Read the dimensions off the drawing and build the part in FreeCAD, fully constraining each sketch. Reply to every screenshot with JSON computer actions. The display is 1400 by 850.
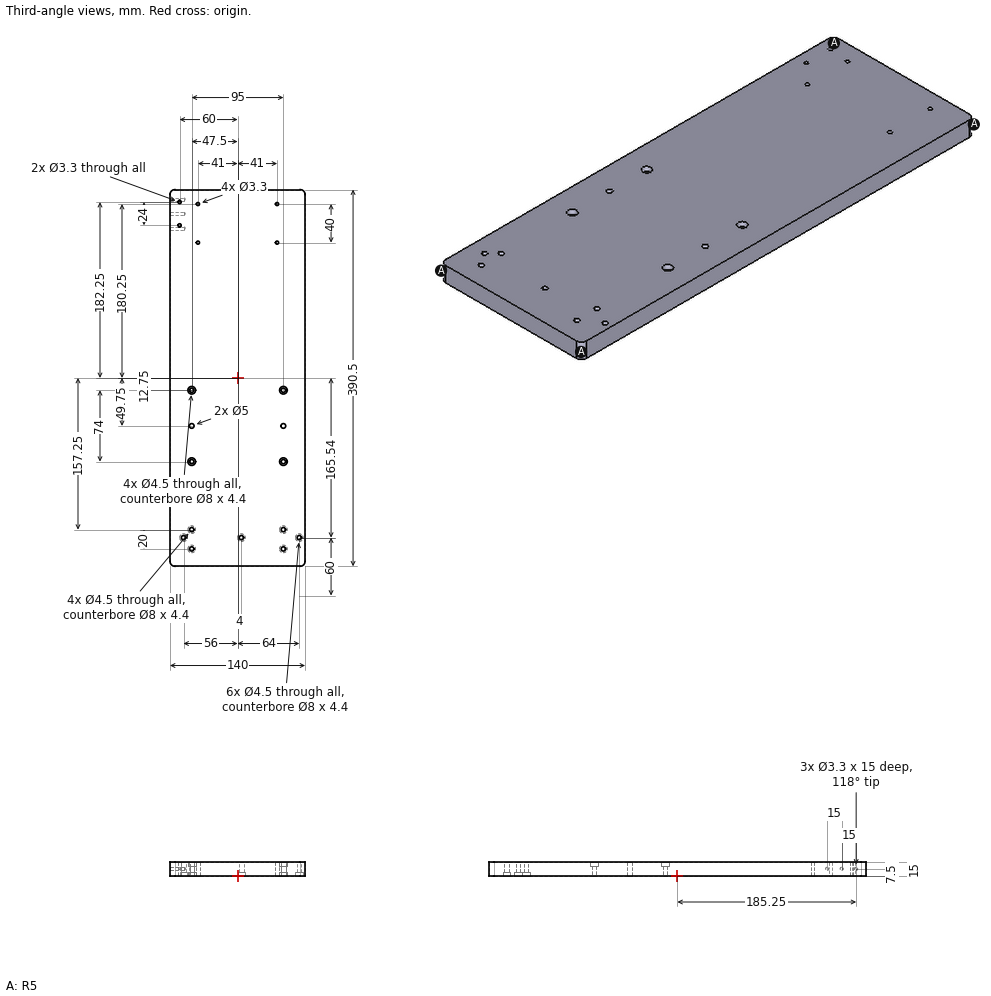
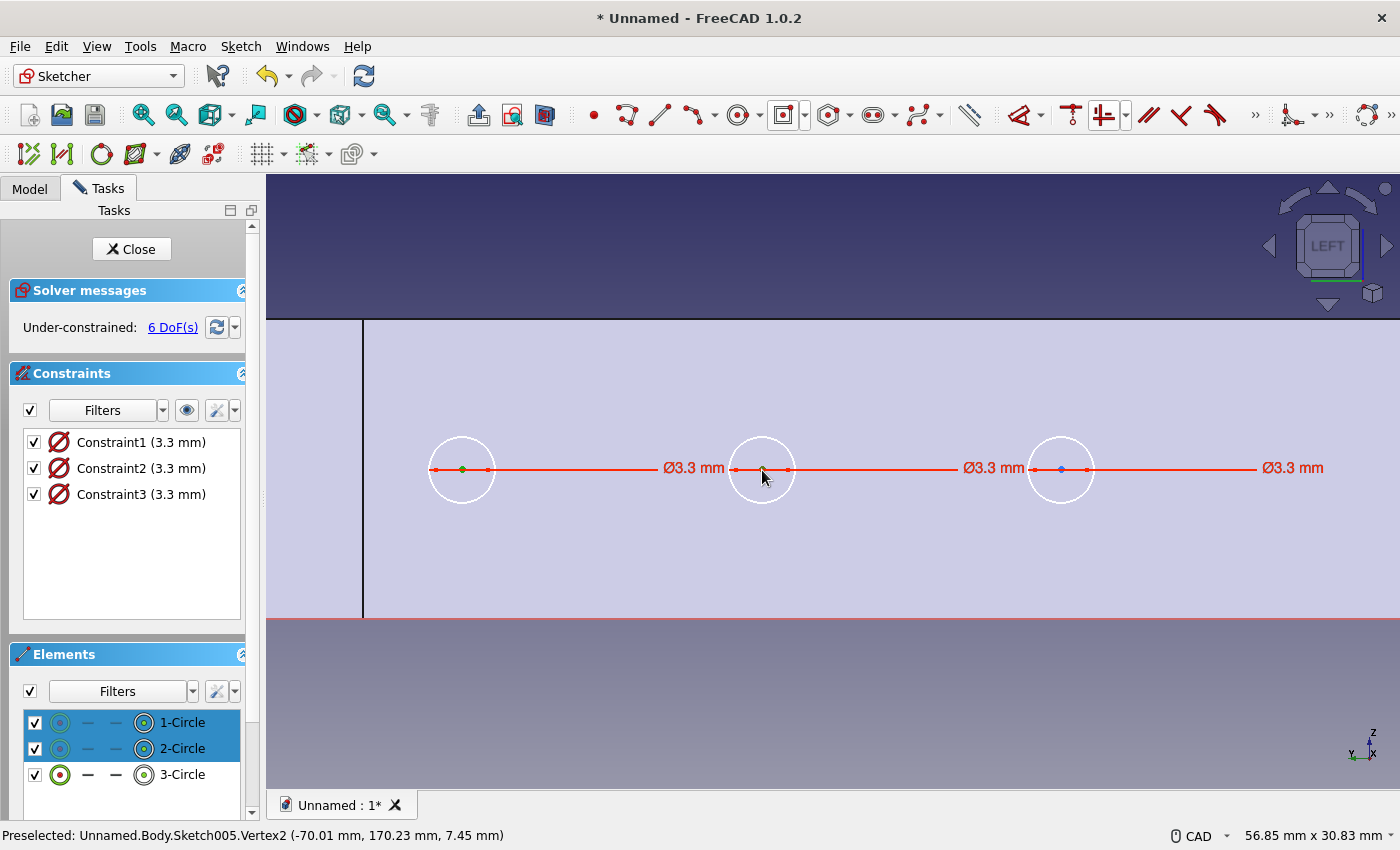
{"action": "key", "text": "h"}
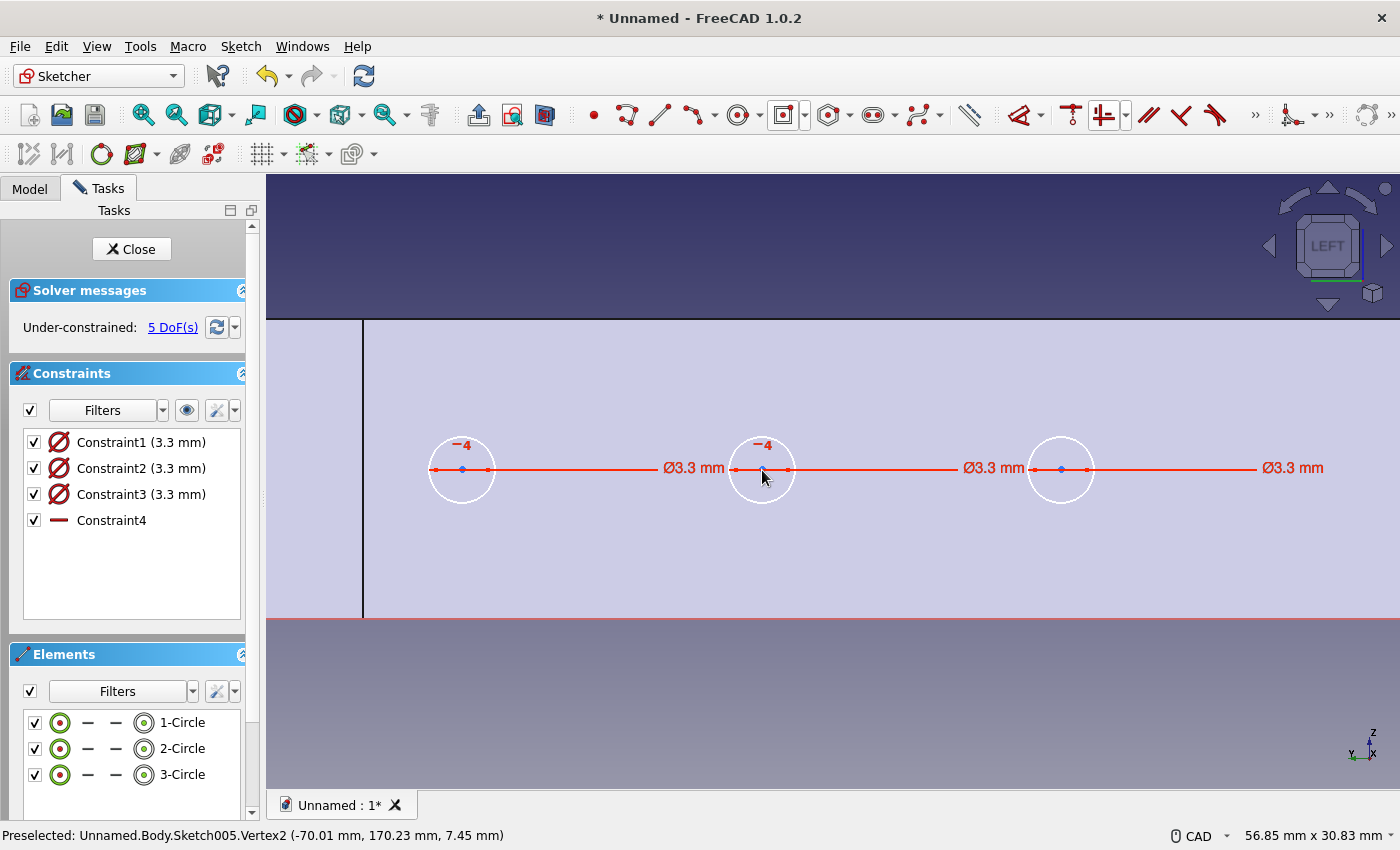
{"action": "left_click", "coordinate": [762, 470]}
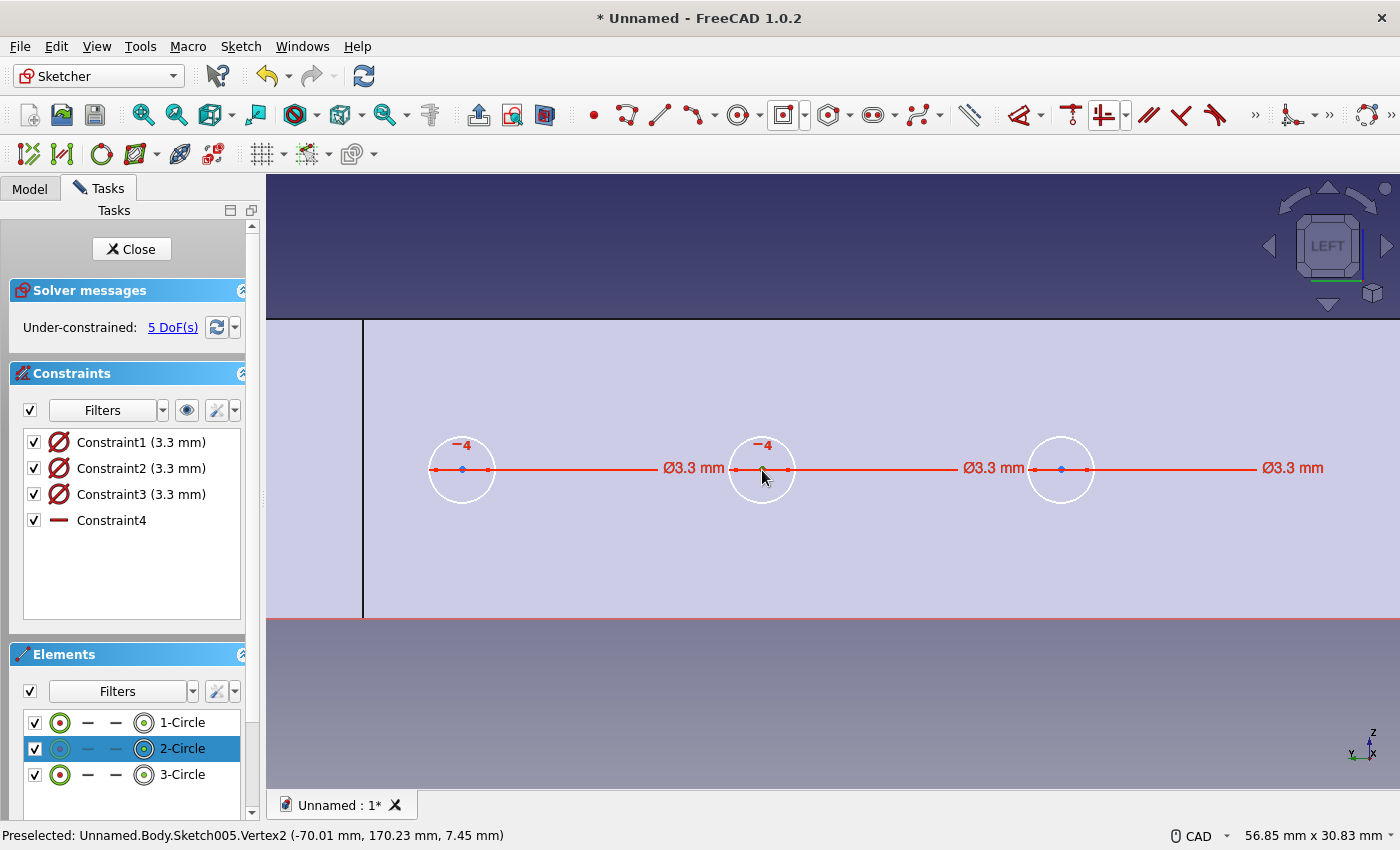
{"action": "left_click", "coordinate": [1061, 470]}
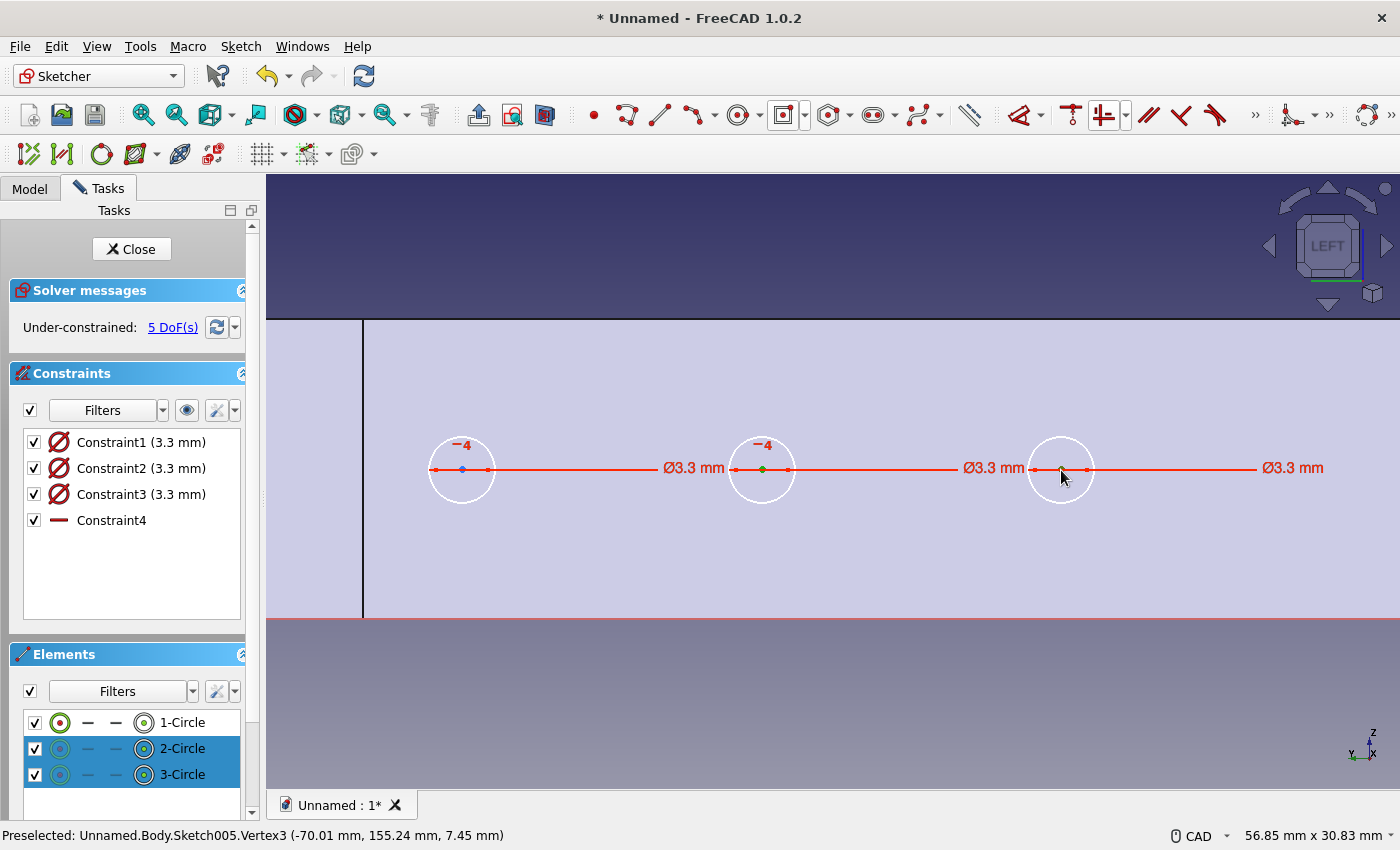
{"action": "key", "text": "h"}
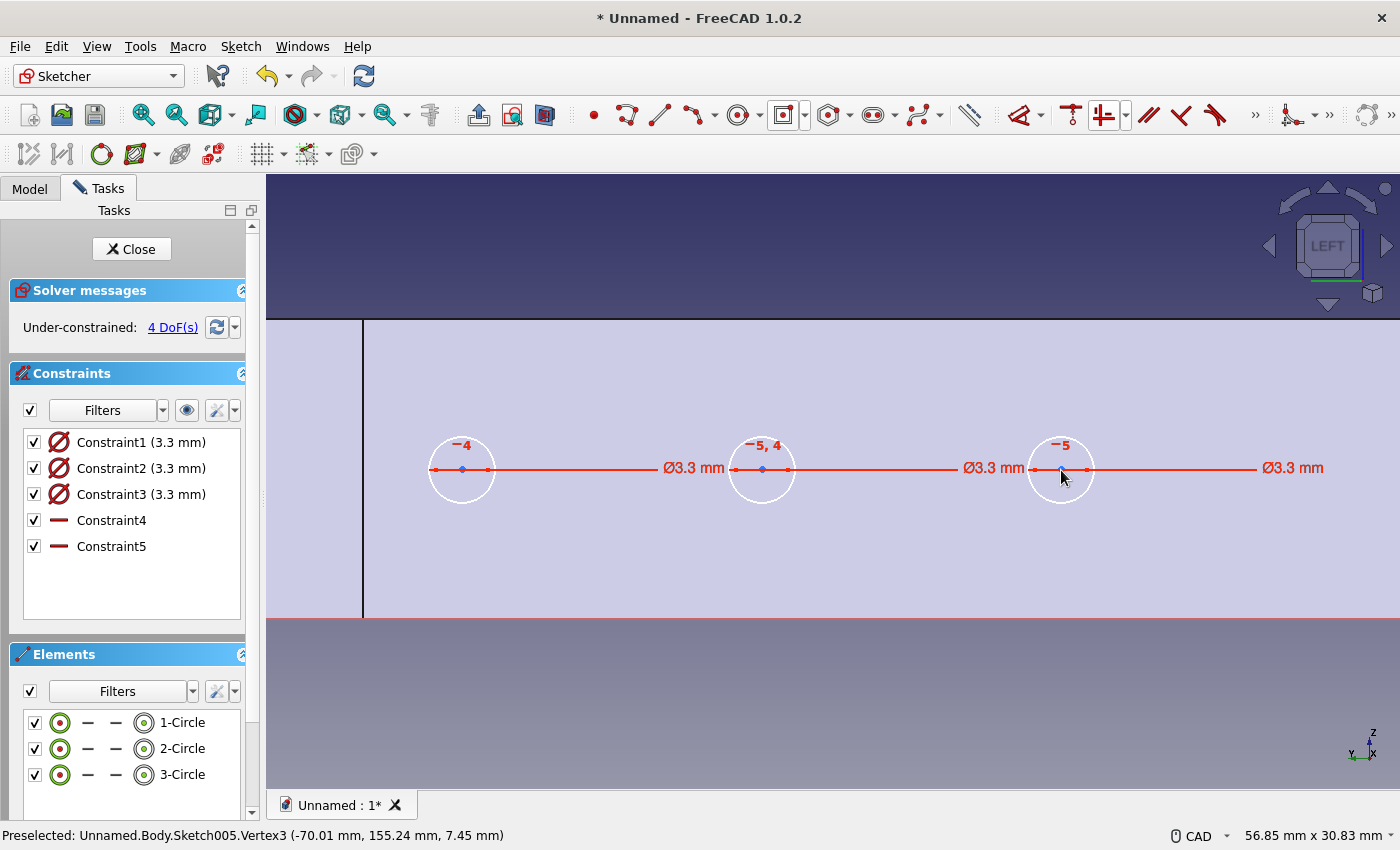
{"action": "left_click", "coordinate": [1018, 116]}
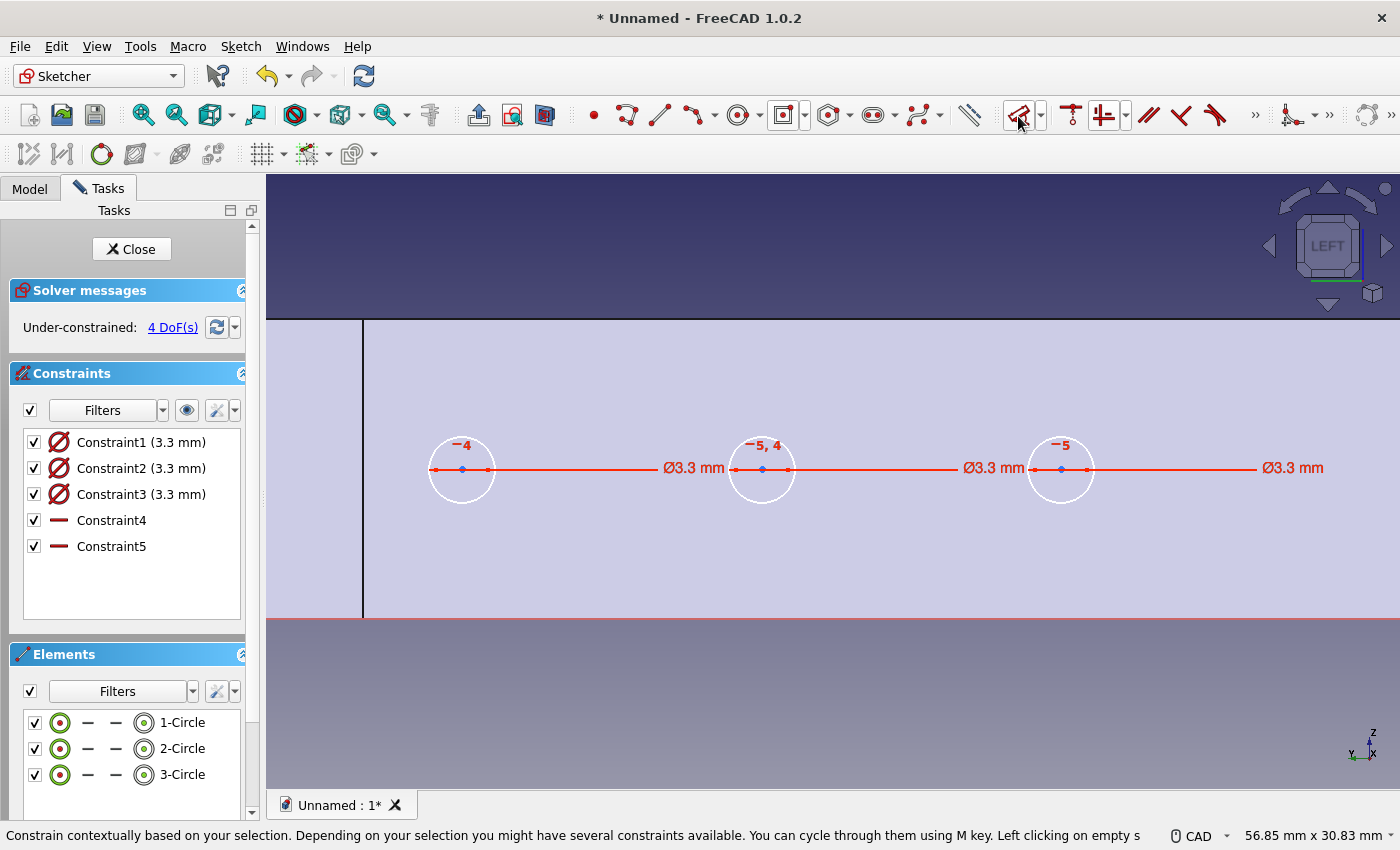
{"action": "left_click", "coordinate": [462, 470]}
{"action": "left_click", "coordinate": [428, 544]}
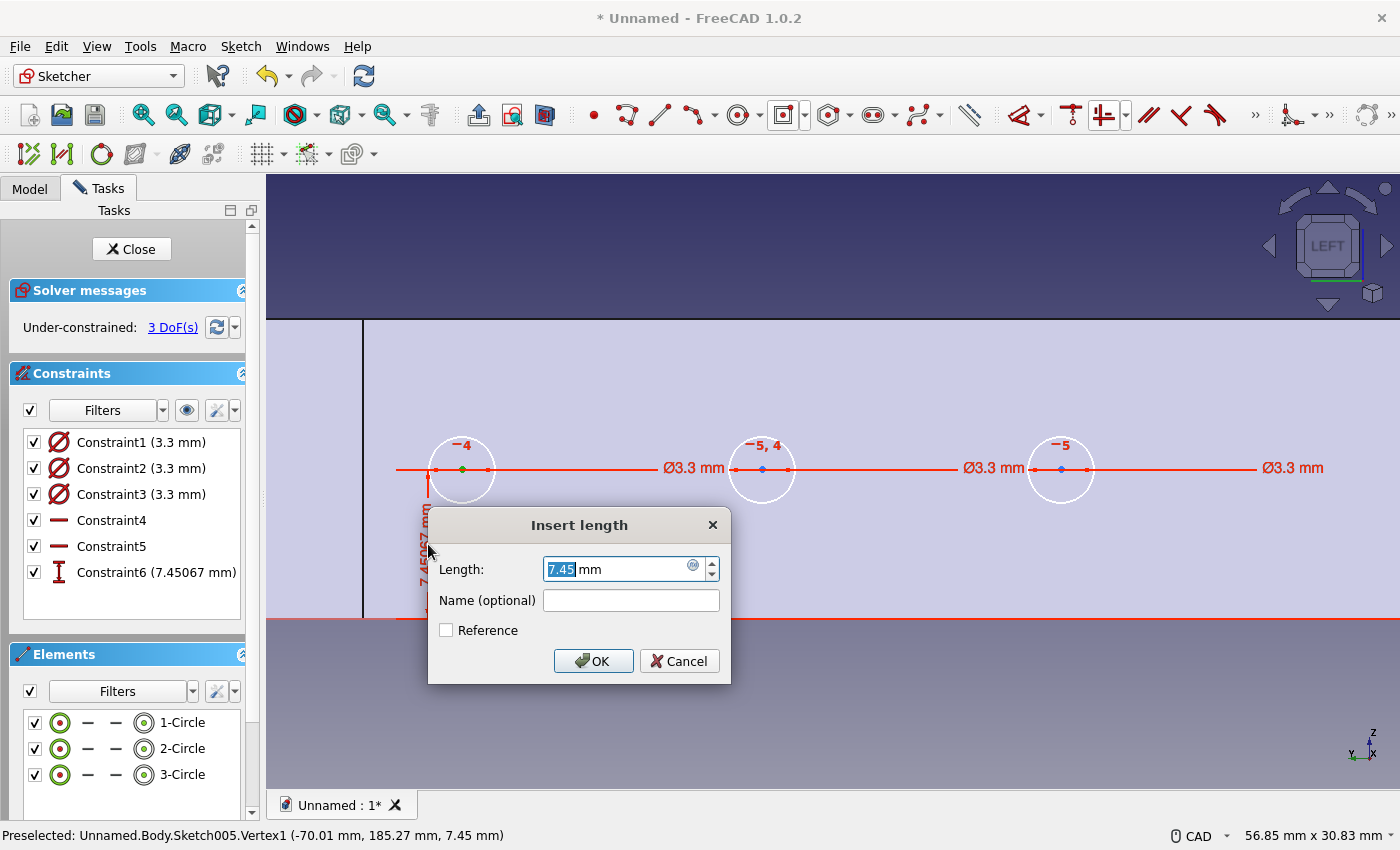
{"action": "type", "text": "7.5"}
{"action": "key", "text": "Return"}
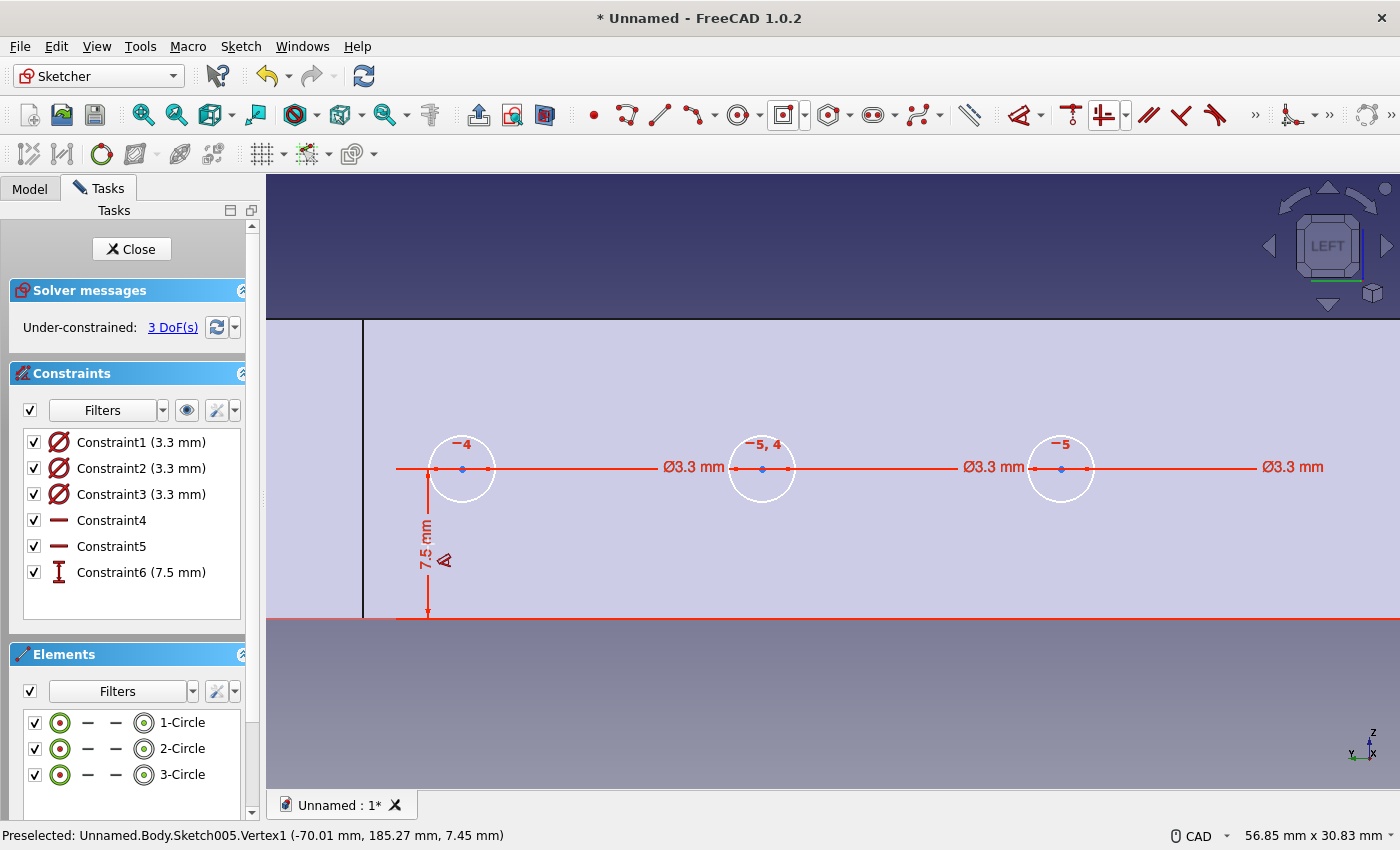
{"action": "left_click", "coordinate": [462, 469]}